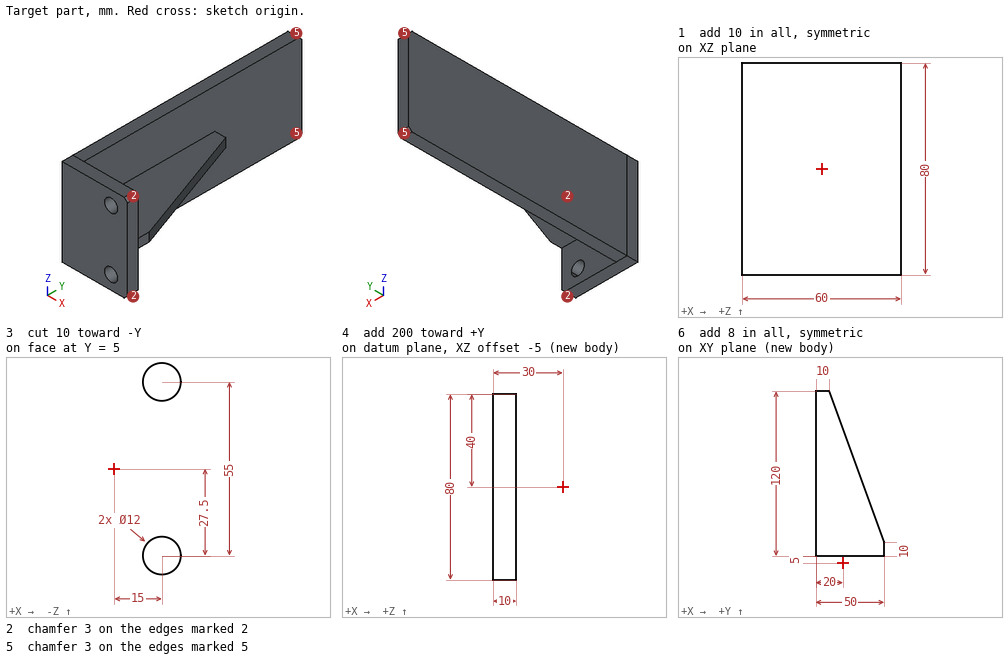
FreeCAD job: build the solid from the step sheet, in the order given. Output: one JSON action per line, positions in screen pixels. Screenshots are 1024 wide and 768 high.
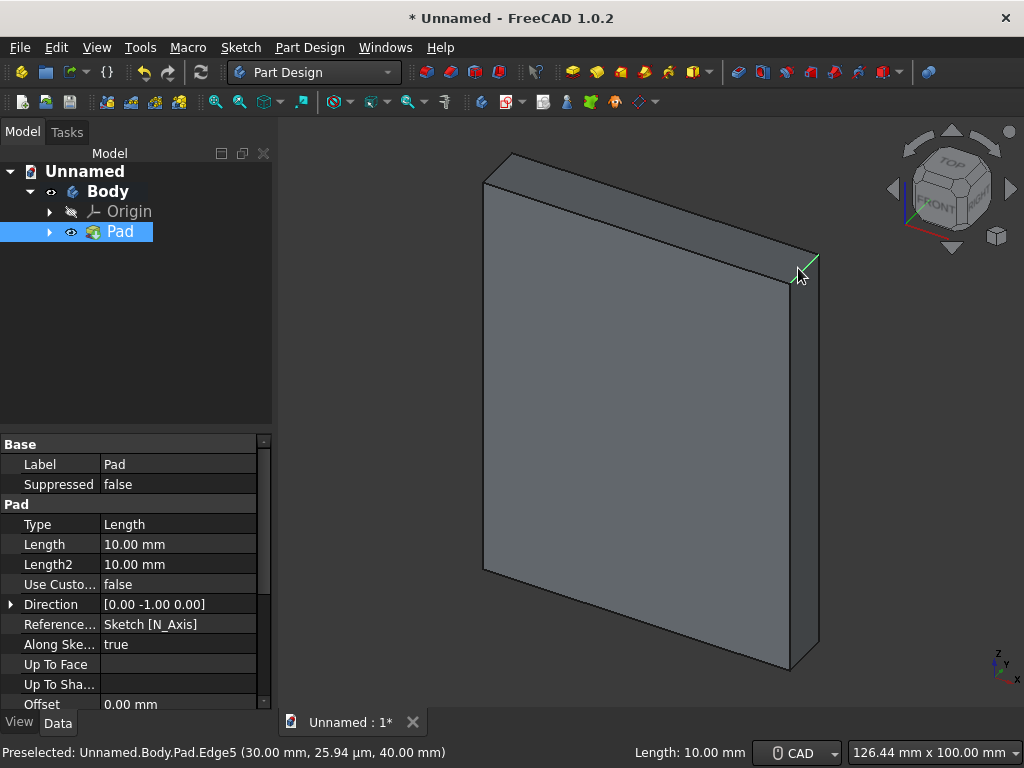
{"action": "key", "text": "0"}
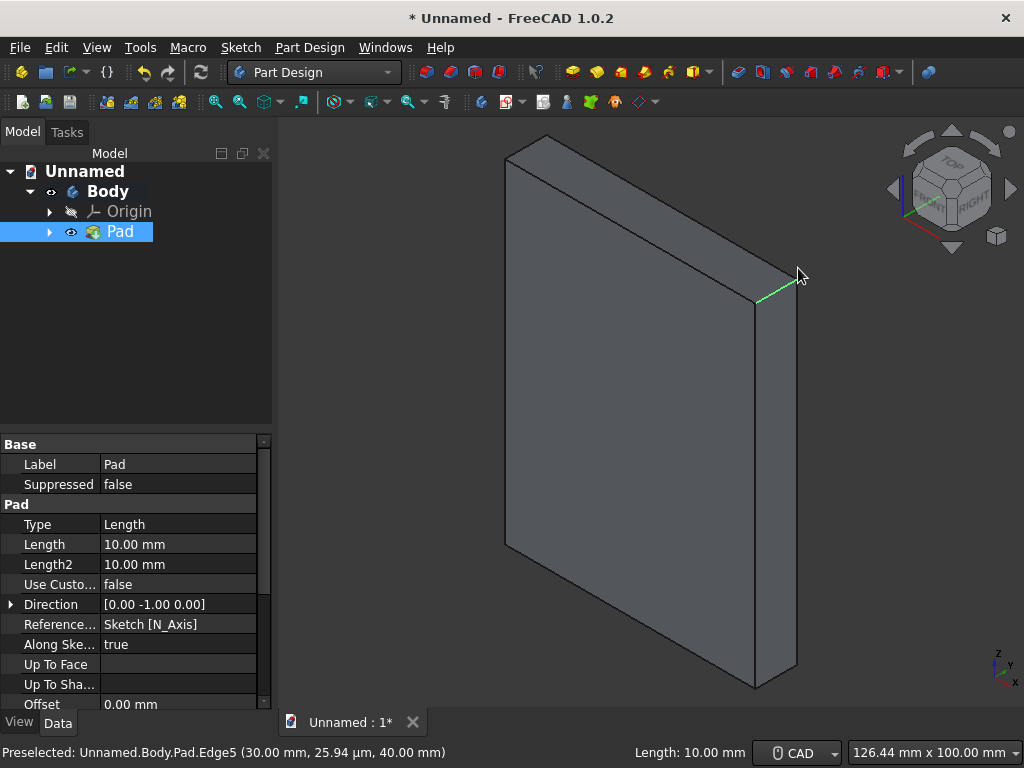
{"action": "key", "text": "2"}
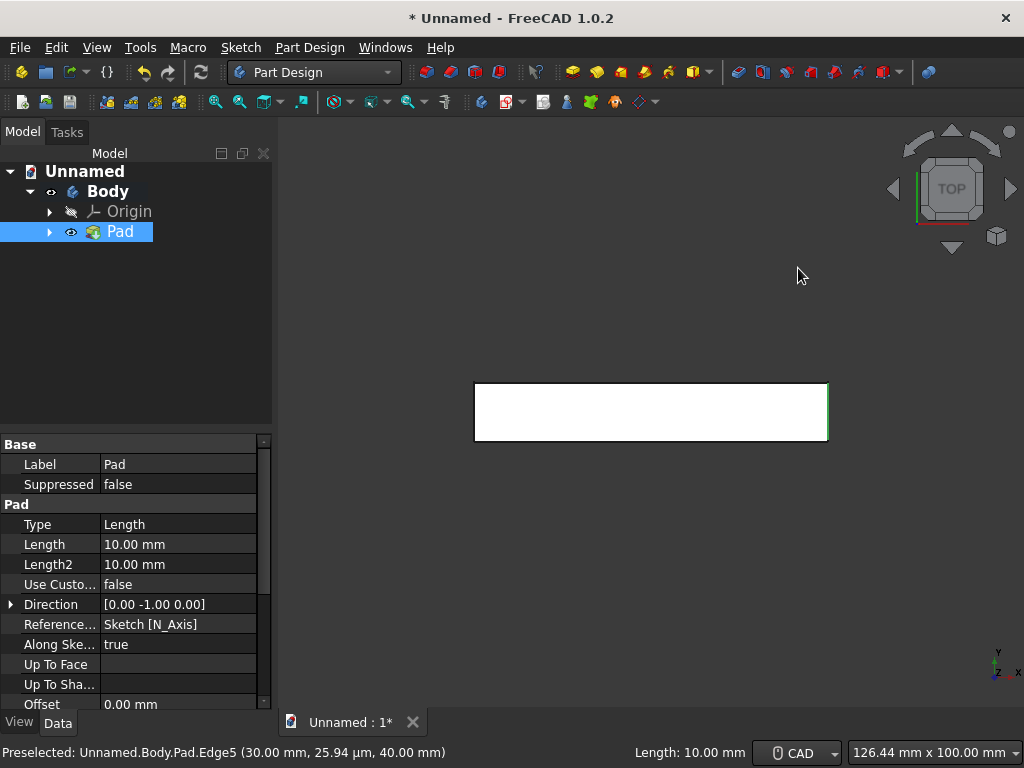
{"action": "key", "text": "1"}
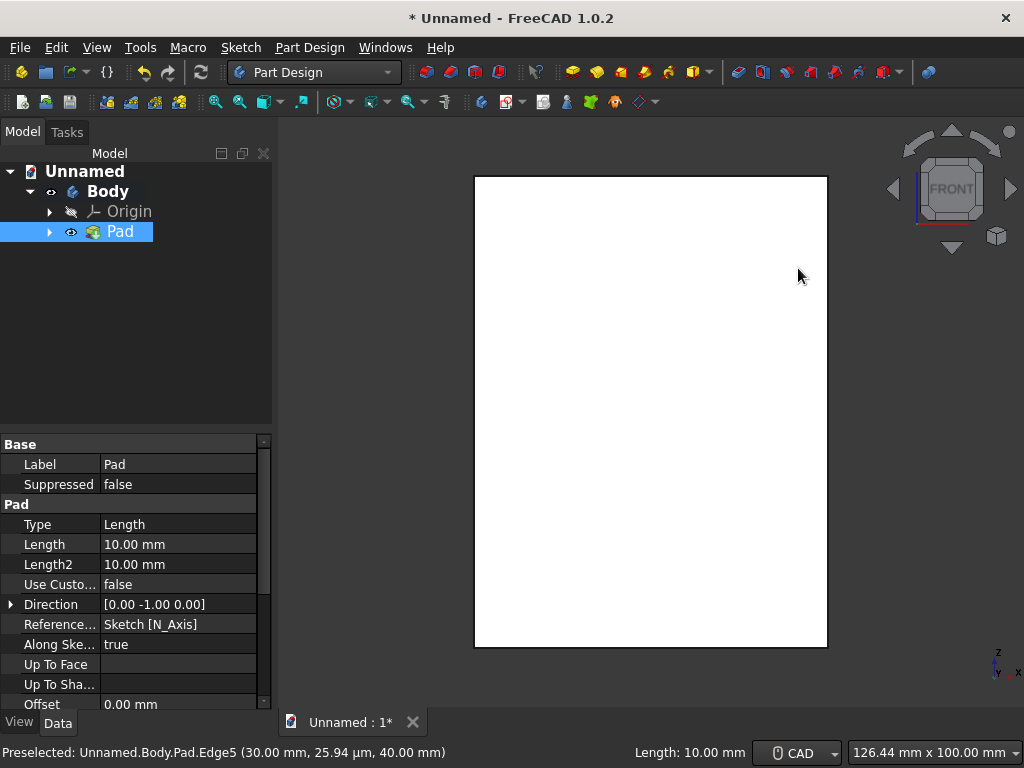
{"action": "key", "text": "3"}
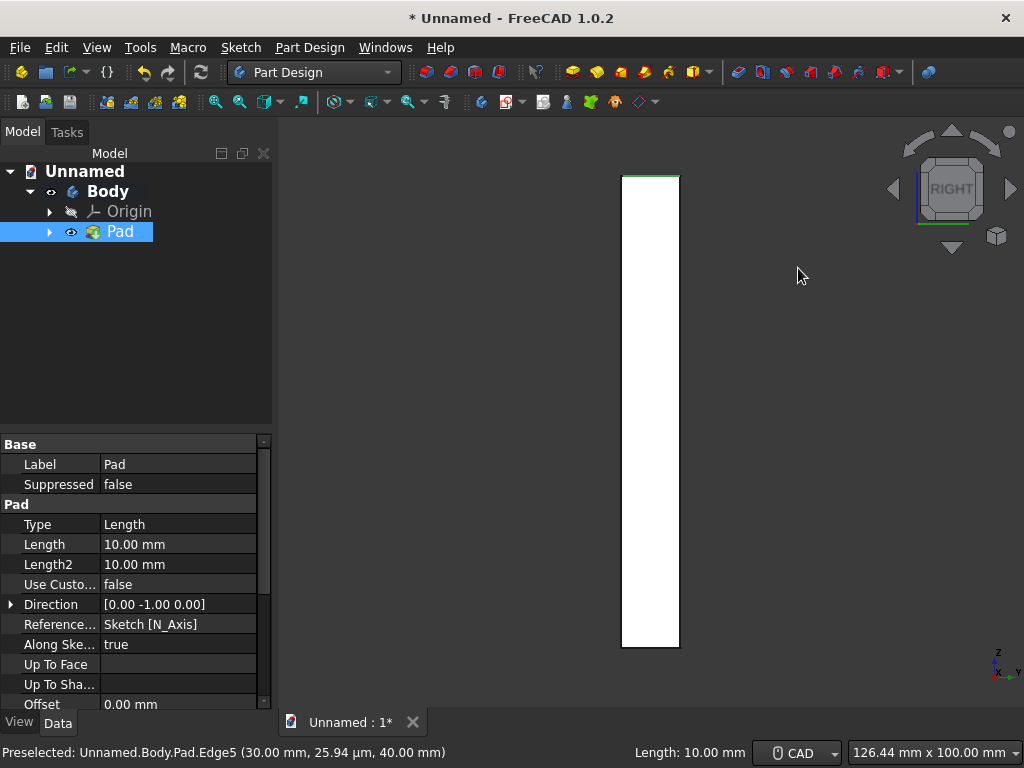
{"action": "left_click", "coordinate": [651, 647], "text": "ctrl"}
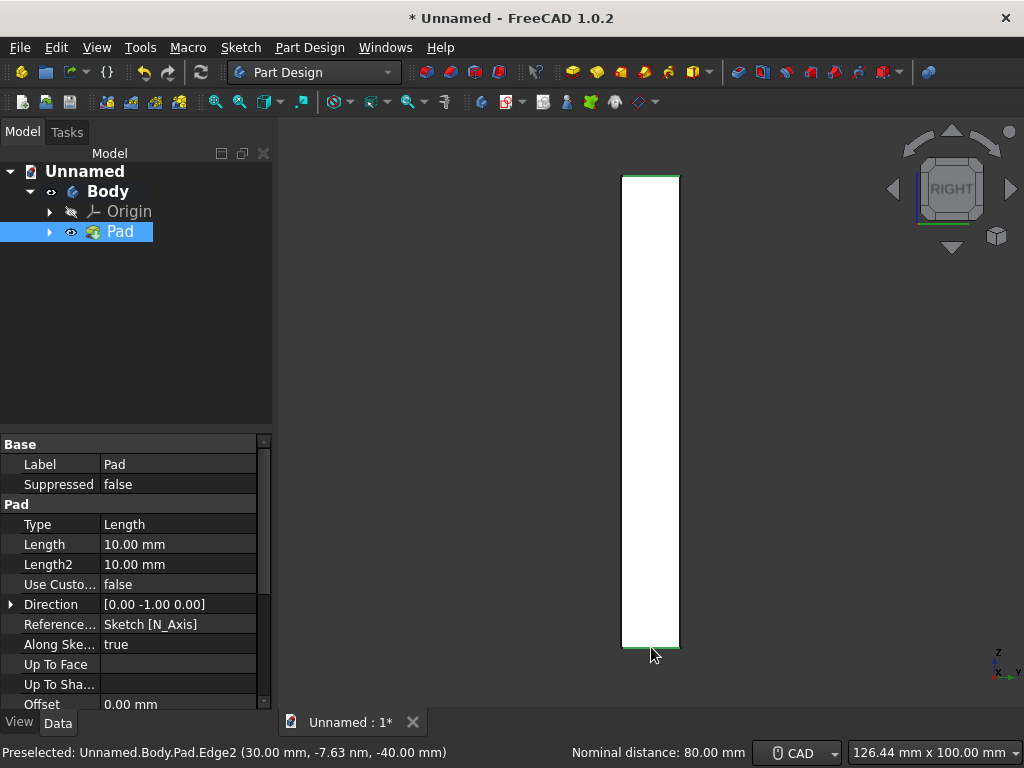
{"action": "left_click", "coordinate": [452, 72]}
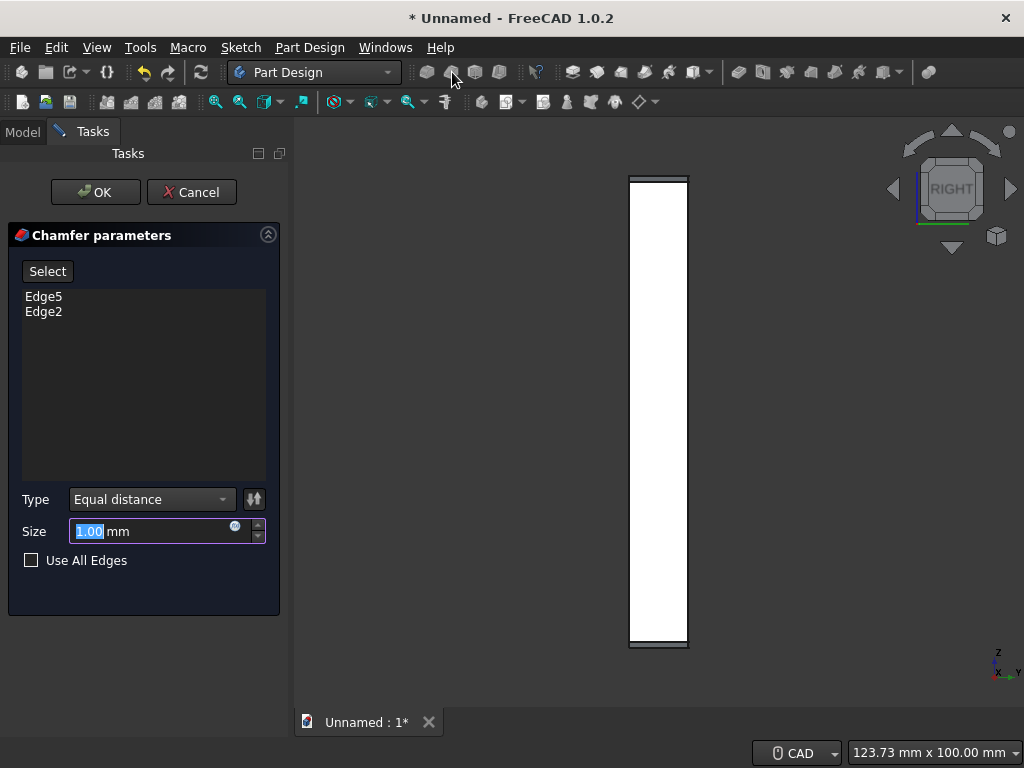
{"action": "type", "text": "3"}
{"action": "key", "text": "Tab"}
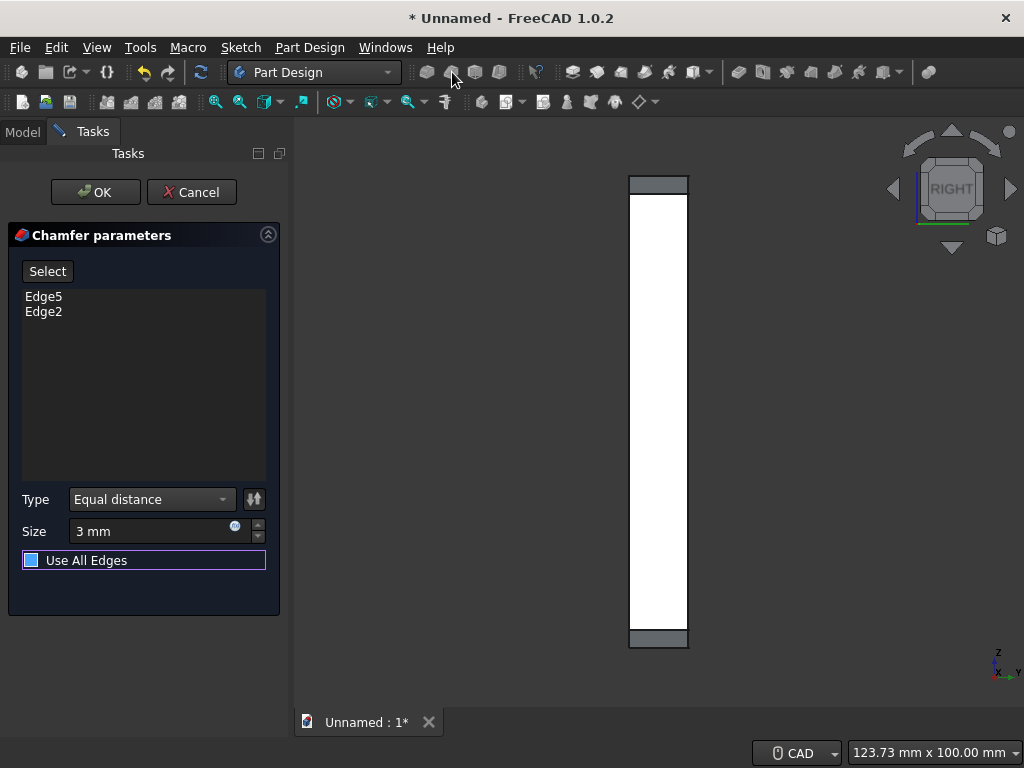
{"action": "left_click", "coordinate": [96, 192]}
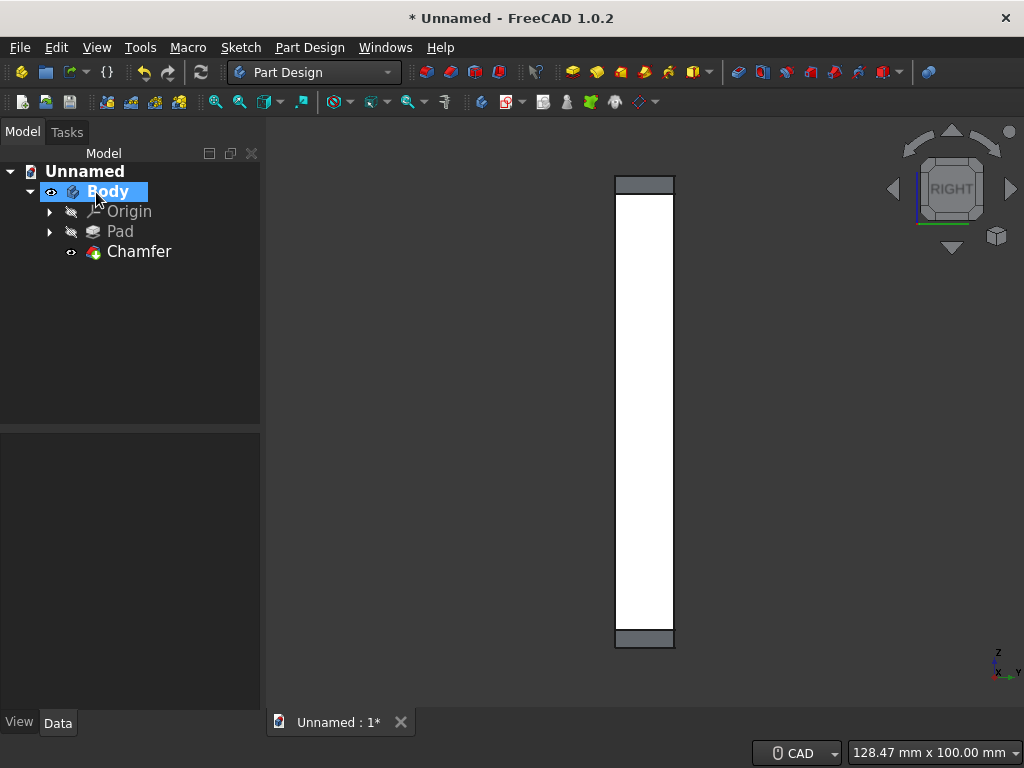
{"action": "key", "text": "4"}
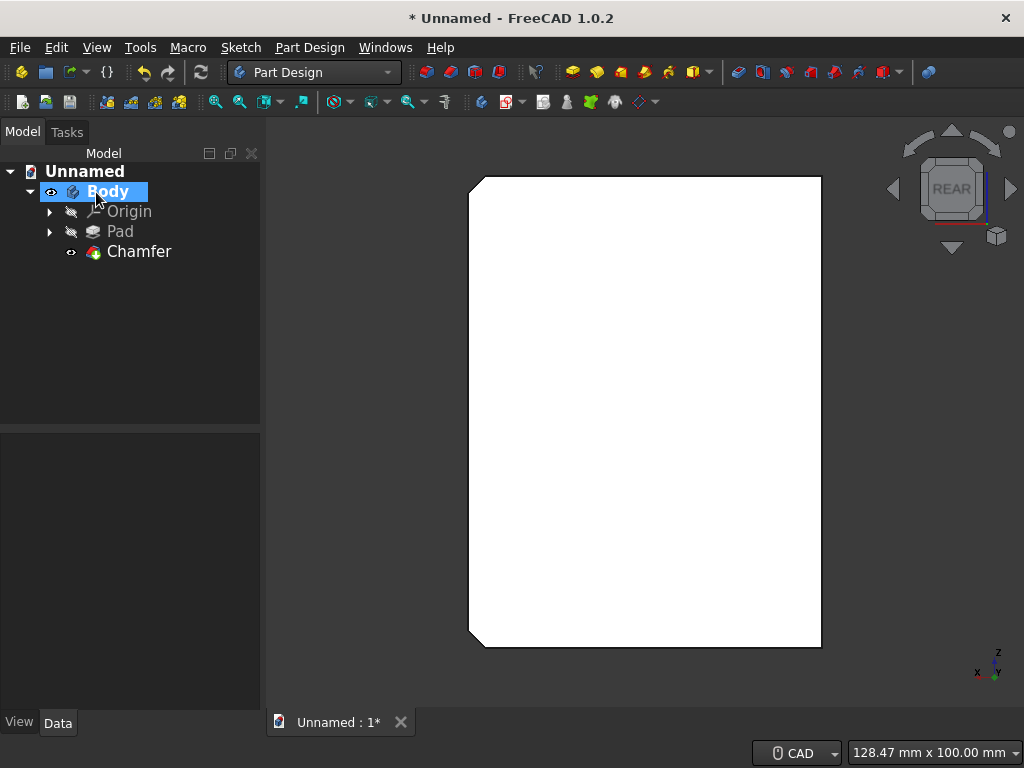
{"action": "left_click", "coordinate": [645, 411]}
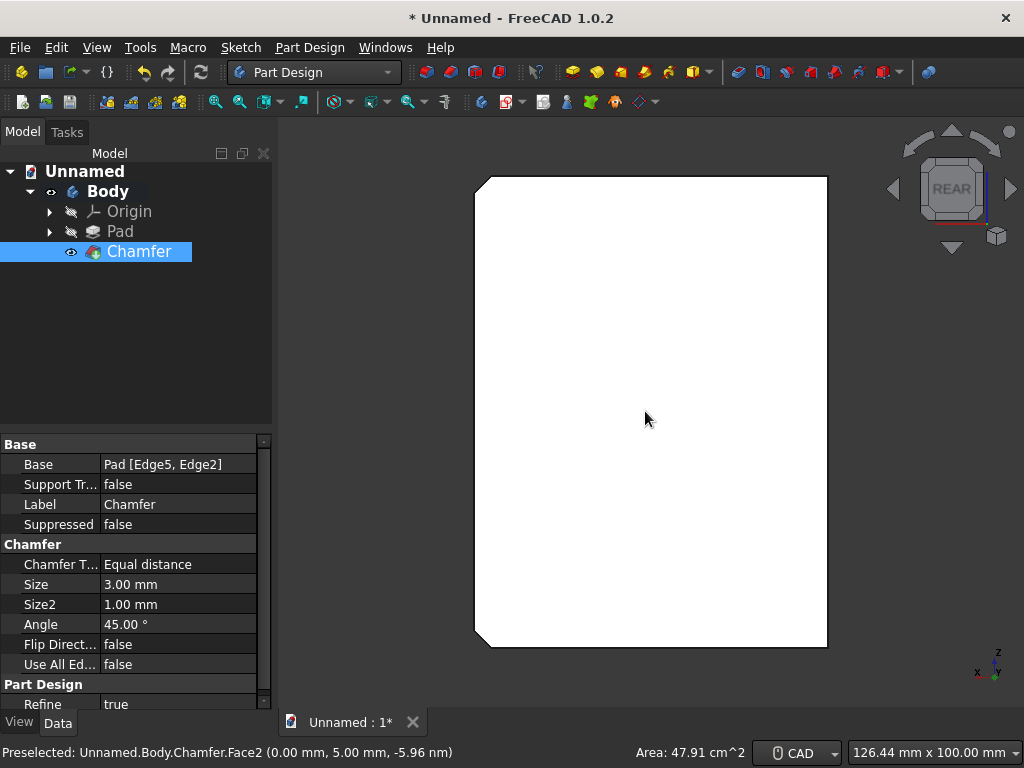
{"action": "left_click", "coordinate": [506, 102]}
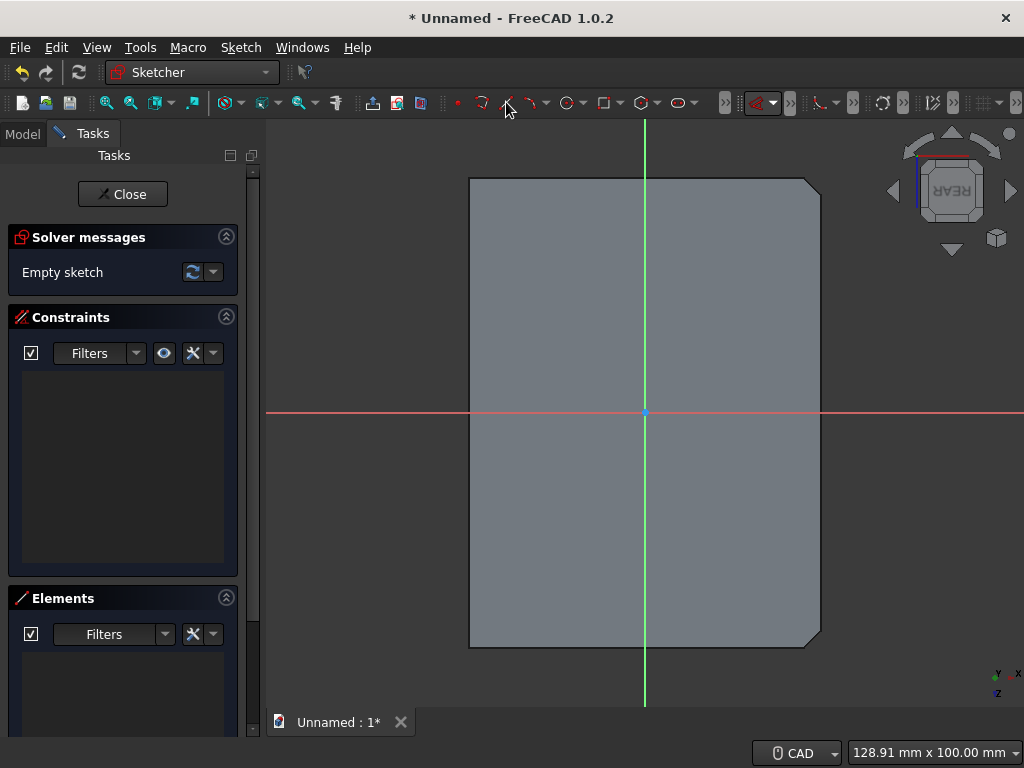
{"action": "left_click", "coordinate": [568, 104]}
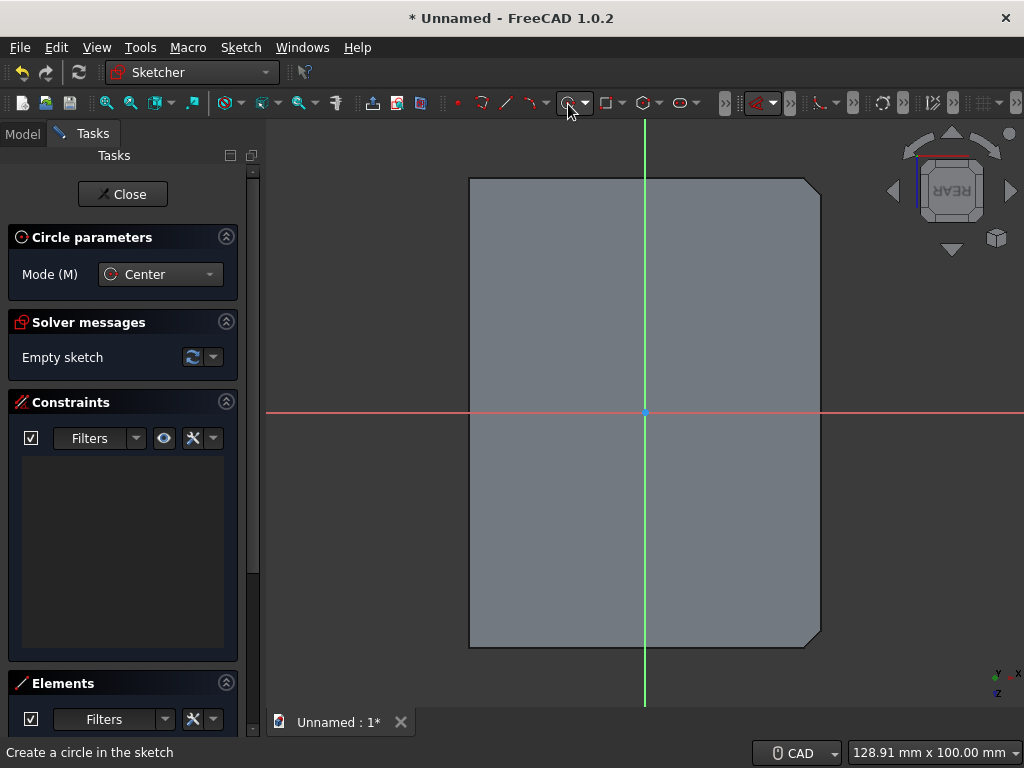
{"action": "left_click", "coordinate": [733, 575]}
{"action": "mouse_move", "coordinate": [758, 550]}